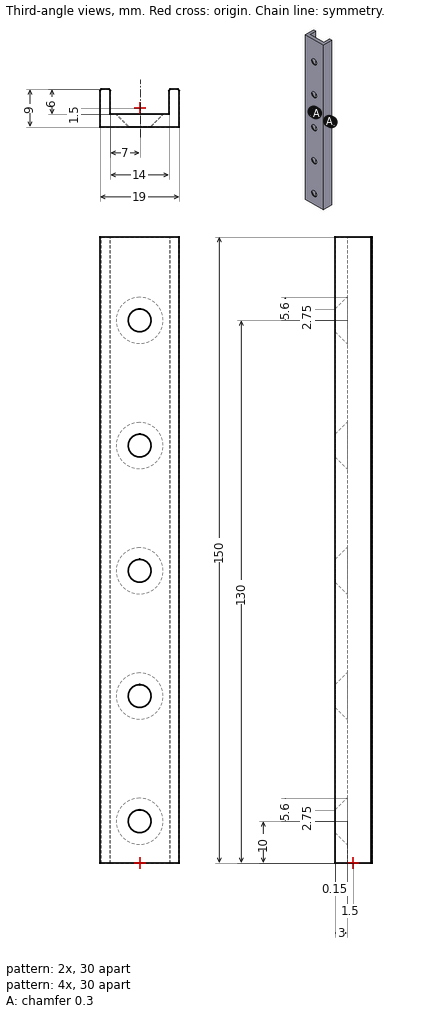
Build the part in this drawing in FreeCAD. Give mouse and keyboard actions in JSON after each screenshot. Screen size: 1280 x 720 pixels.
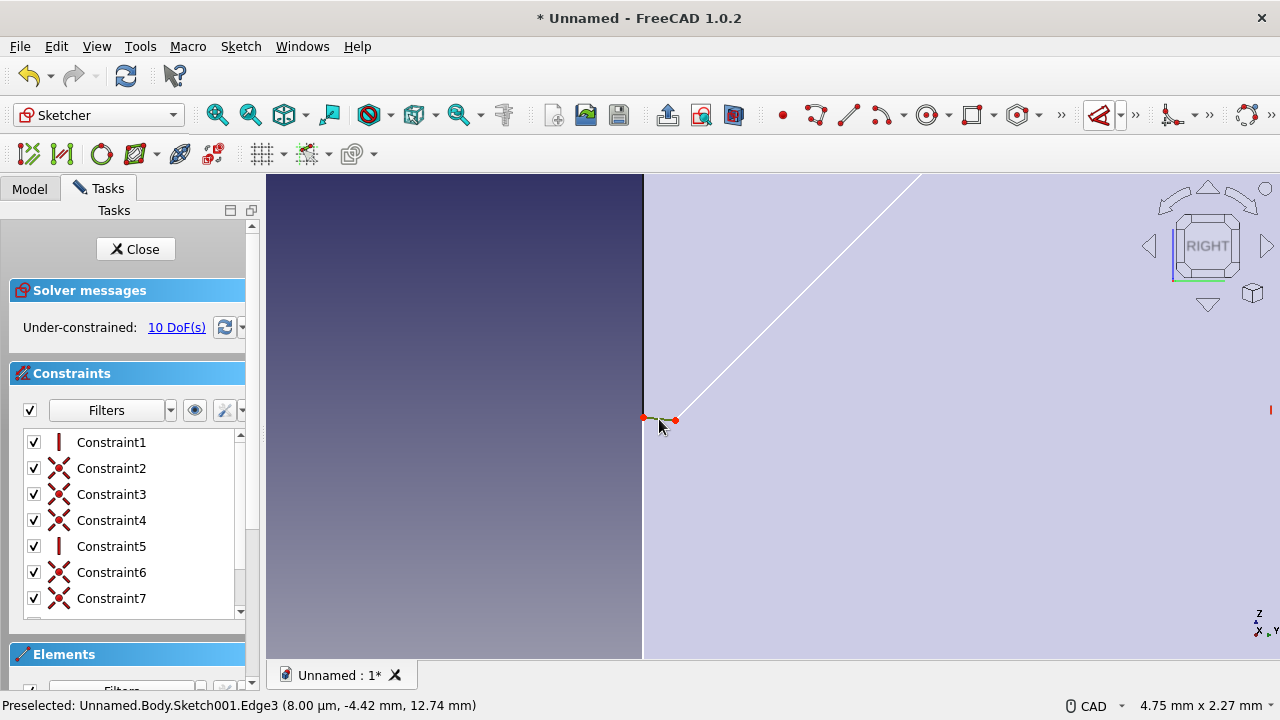
{"action": "key", "text": "h"}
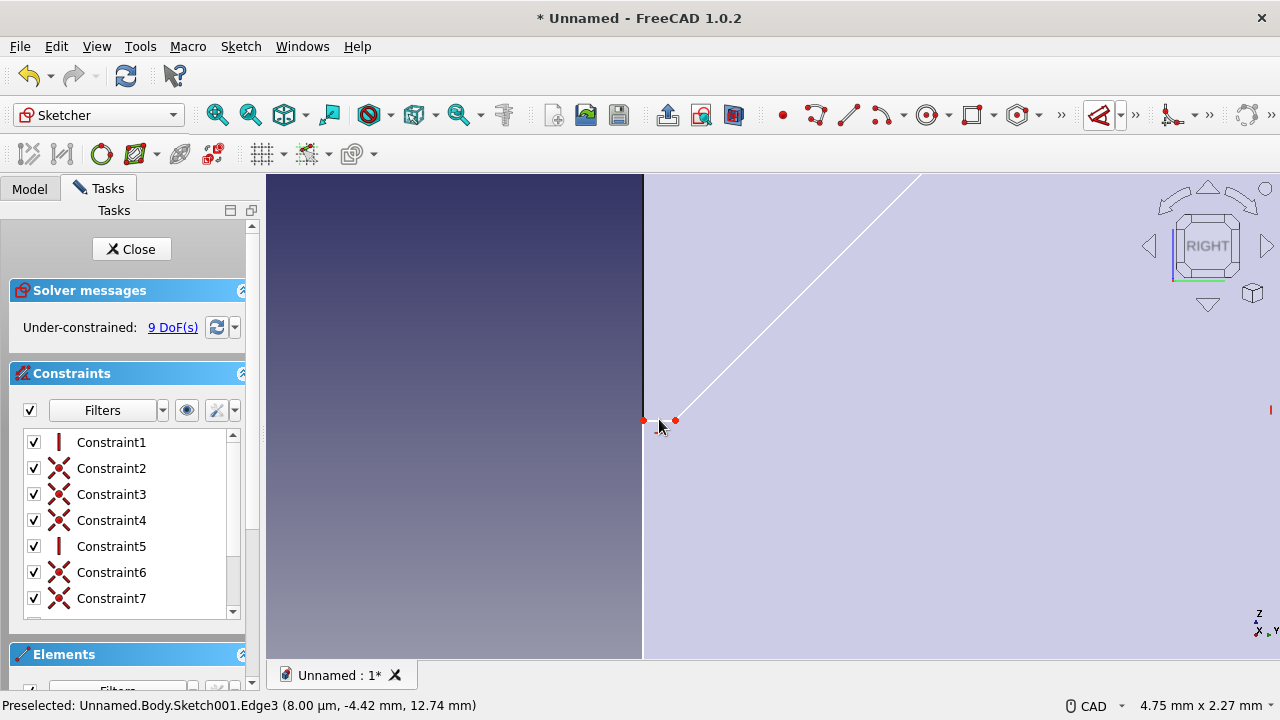
{"action": "scroll", "coordinate": [662, 420], "scroll_direction": "down", "scroll_amount": 7}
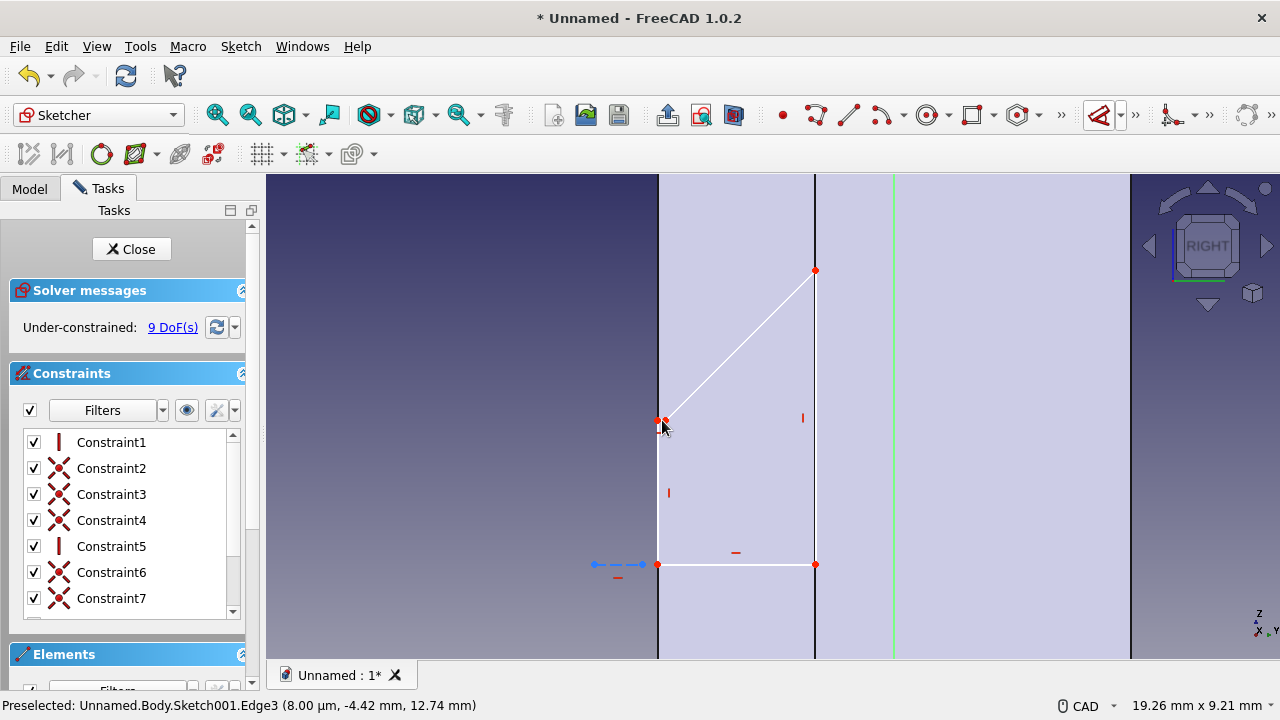
{"action": "left_click", "coordinate": [705, 565]}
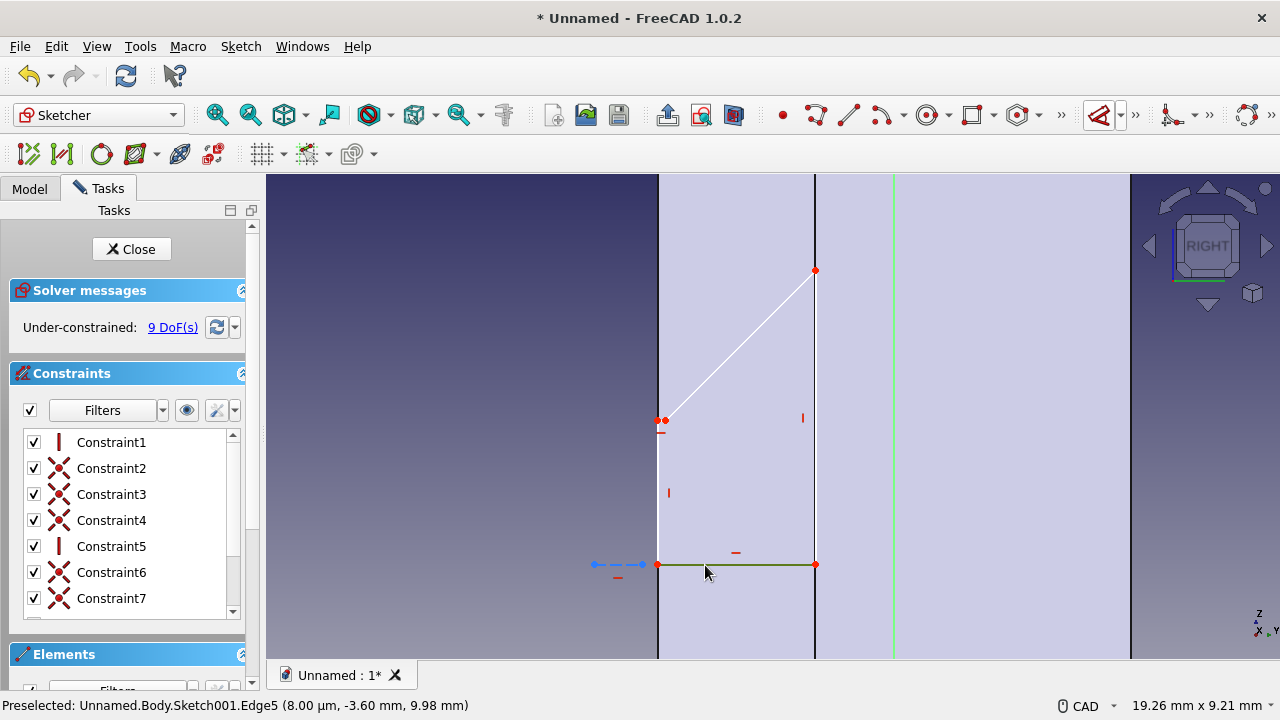
{"action": "left_click", "coordinate": [1120, 116]}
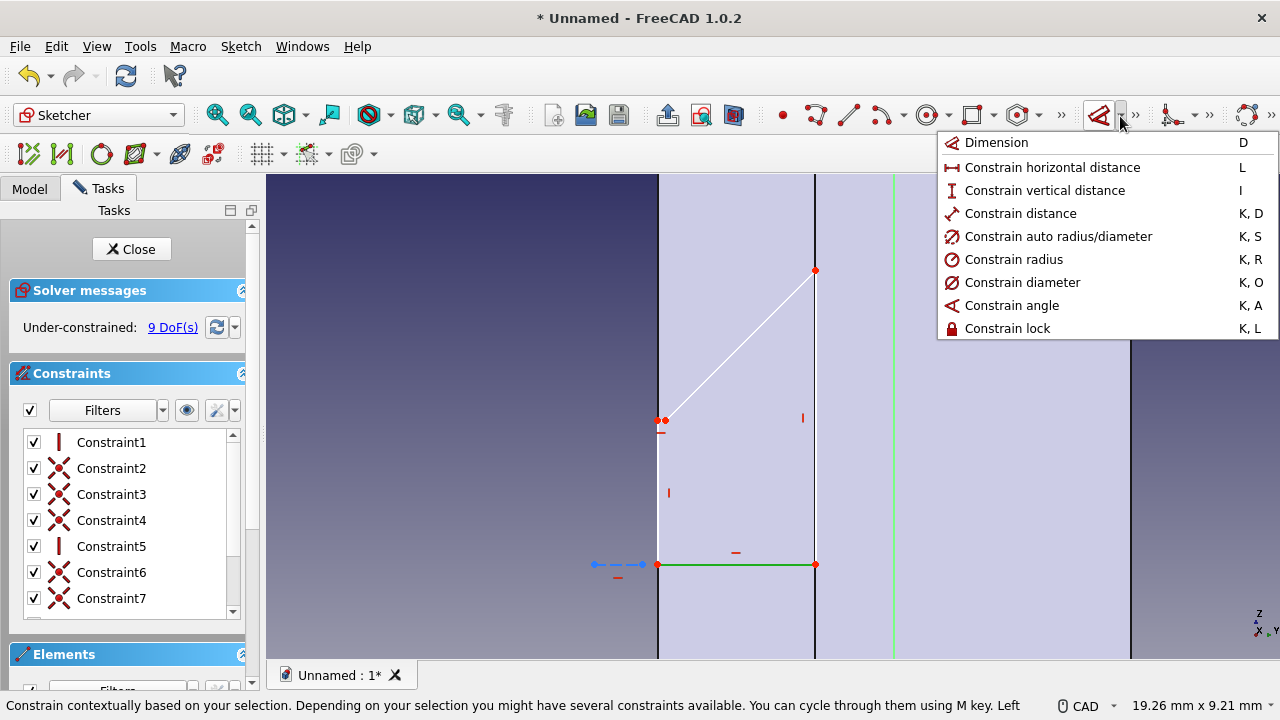
{"action": "left_click", "coordinate": [1108, 168]}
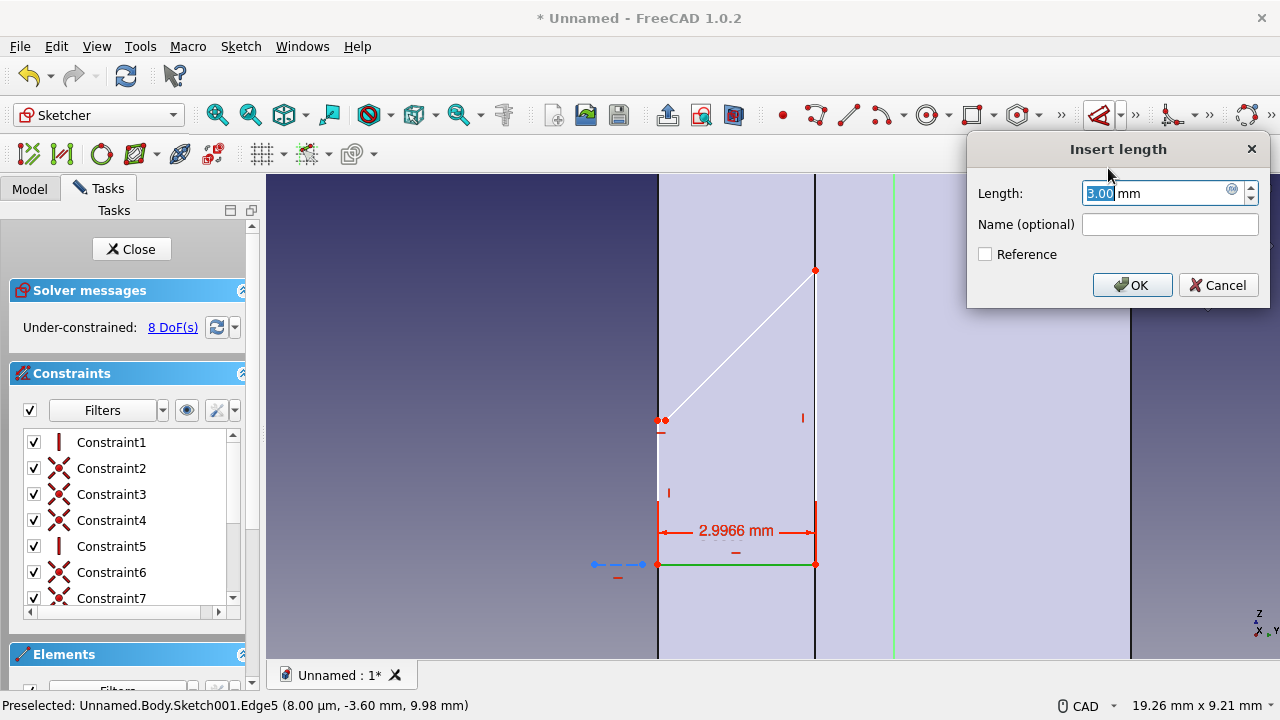
{"action": "type", "text": "3"}
{"action": "key", "text": "Return"}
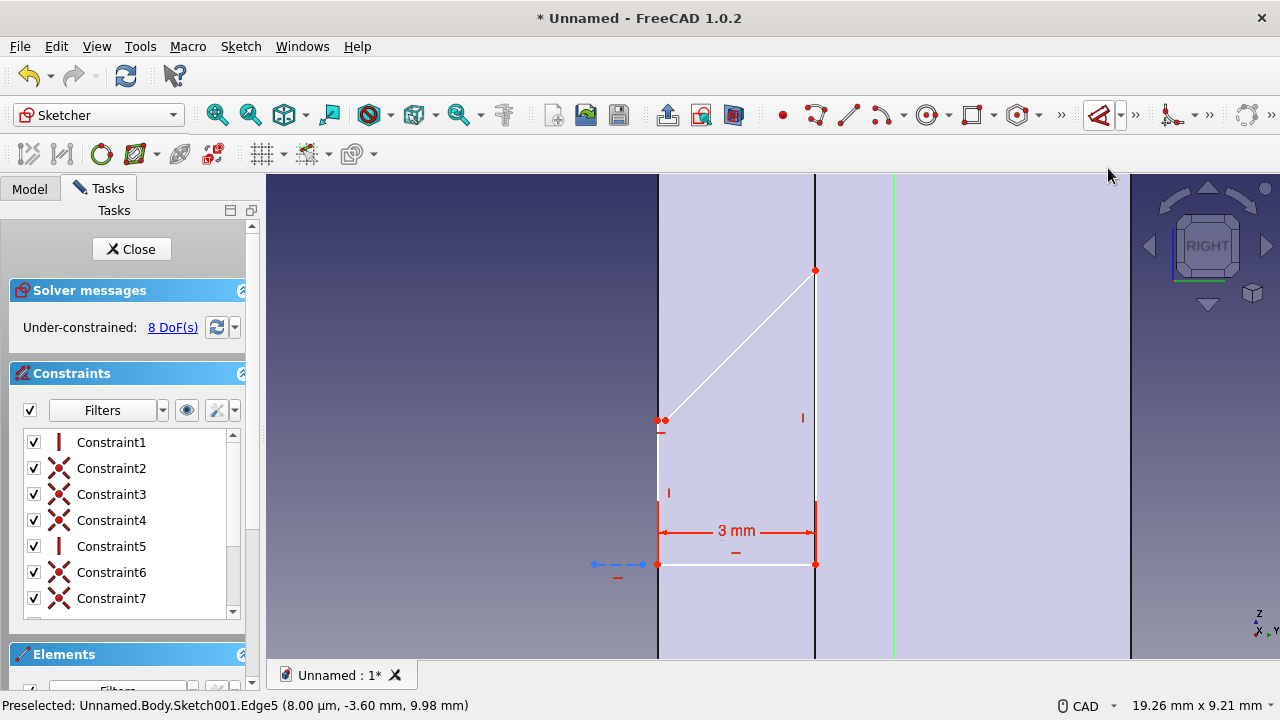
{"action": "left_click", "coordinate": [816, 477]}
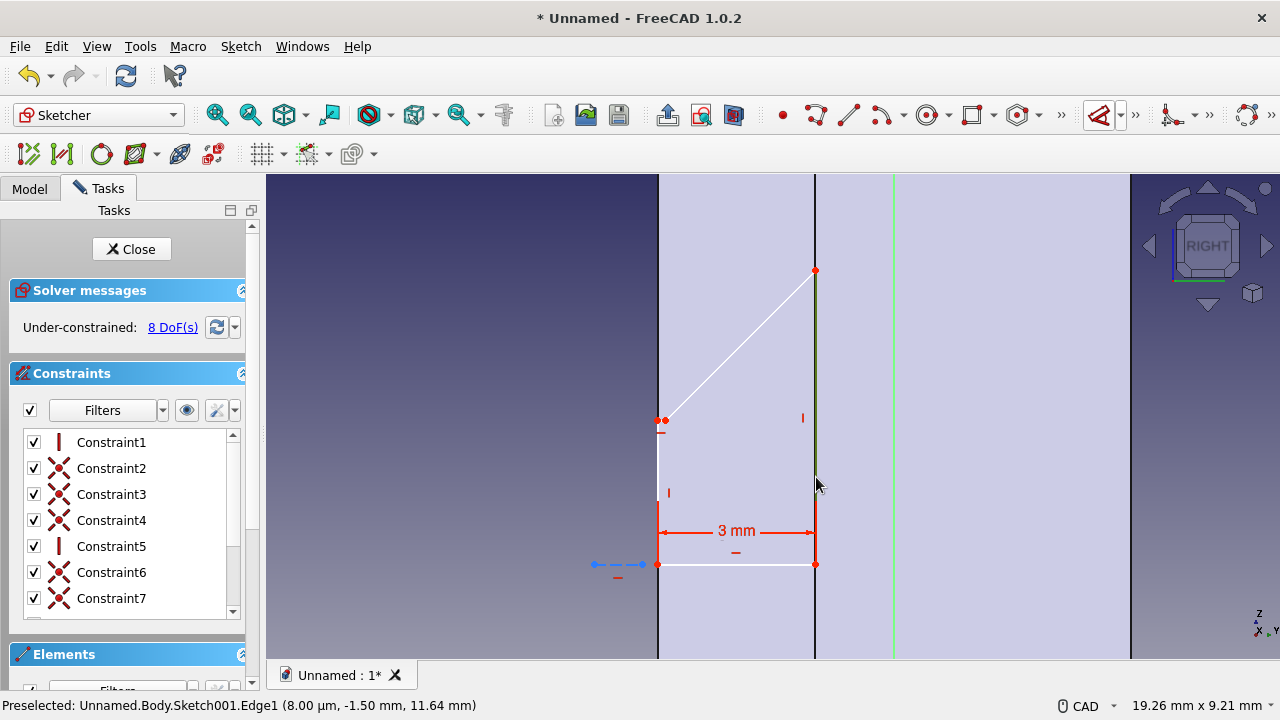
{"action": "left_click", "coordinate": [1120, 116]}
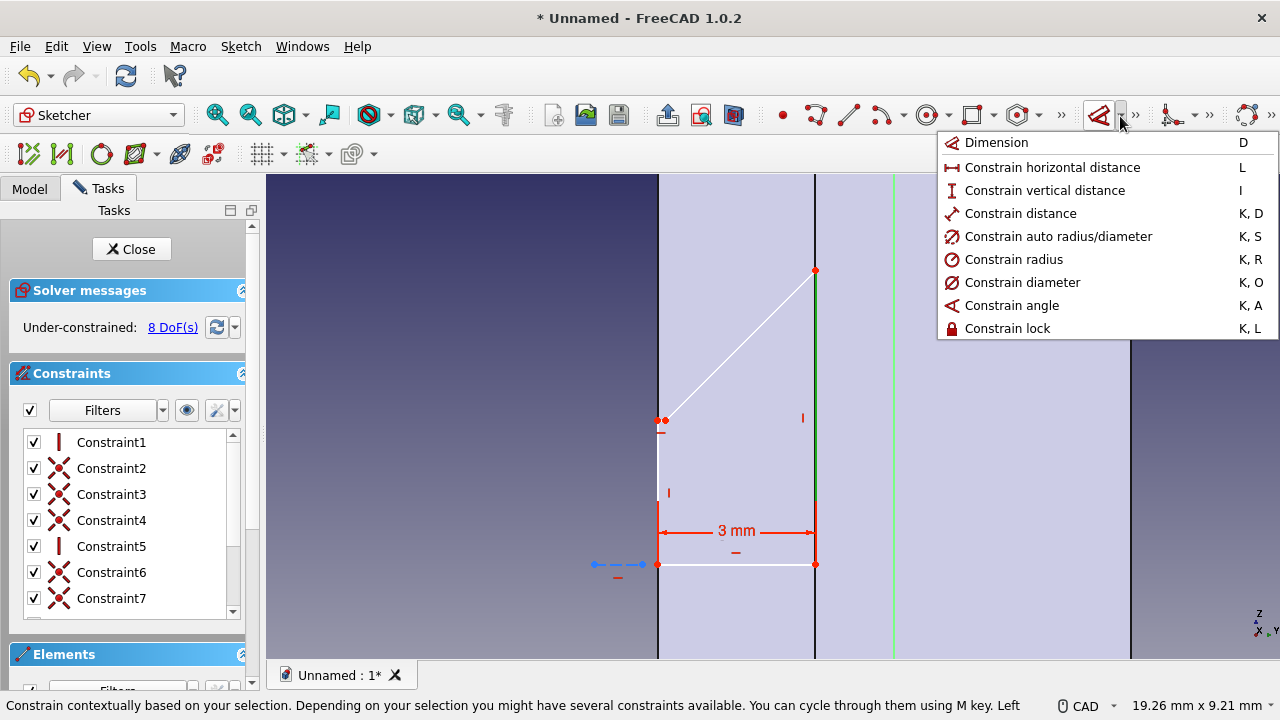
{"action": "left_click", "coordinate": [1108, 190]}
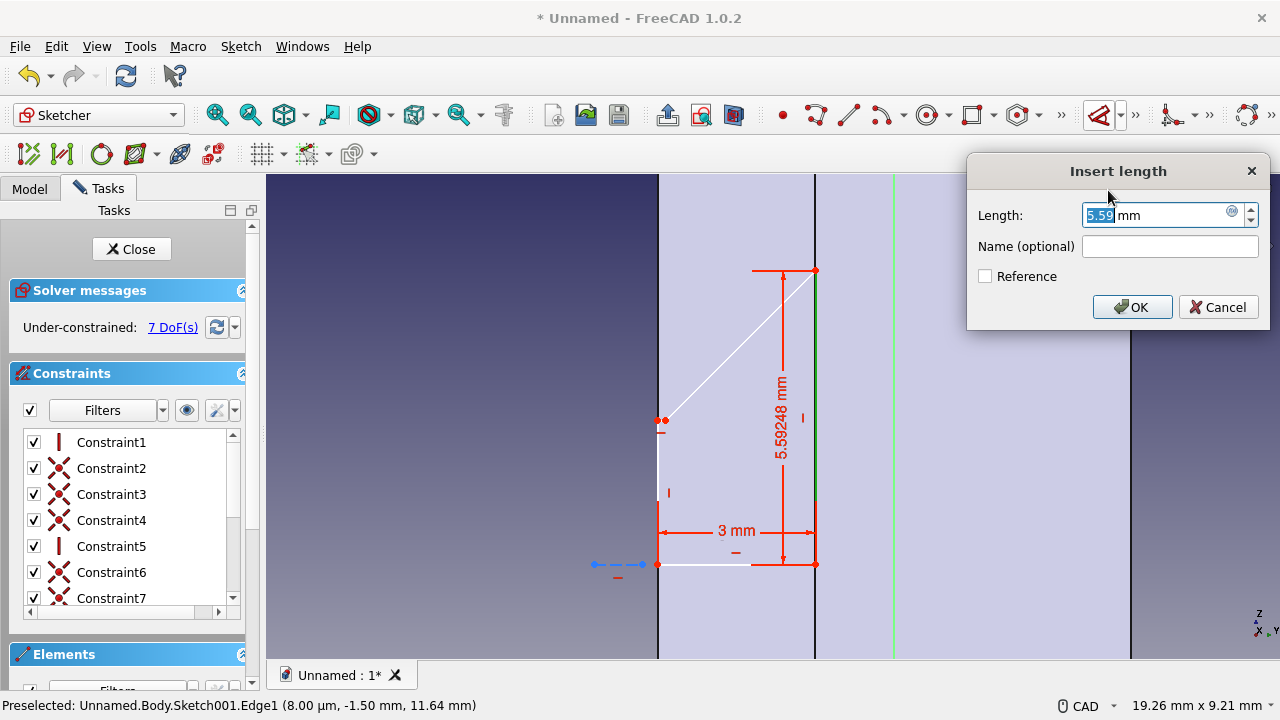
{"action": "type", "text": "5.6"}
{"action": "key", "text": "Return"}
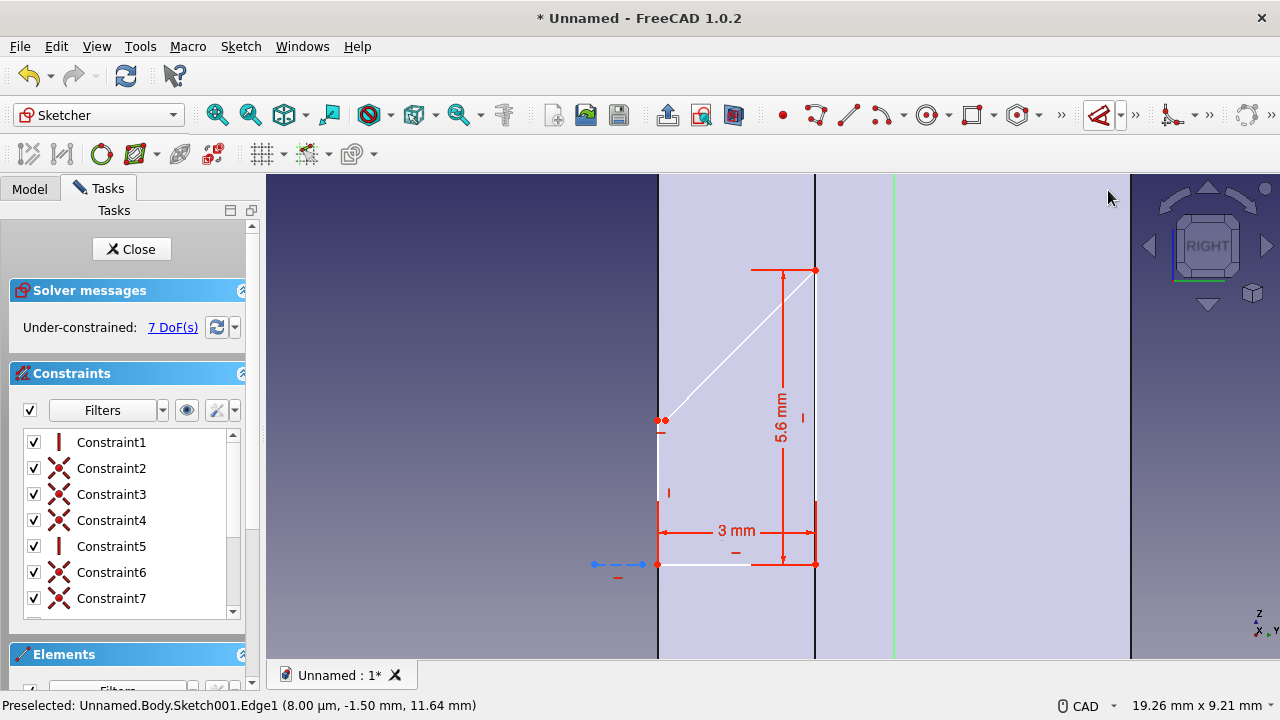
{"action": "left_click", "coordinate": [816, 565]}